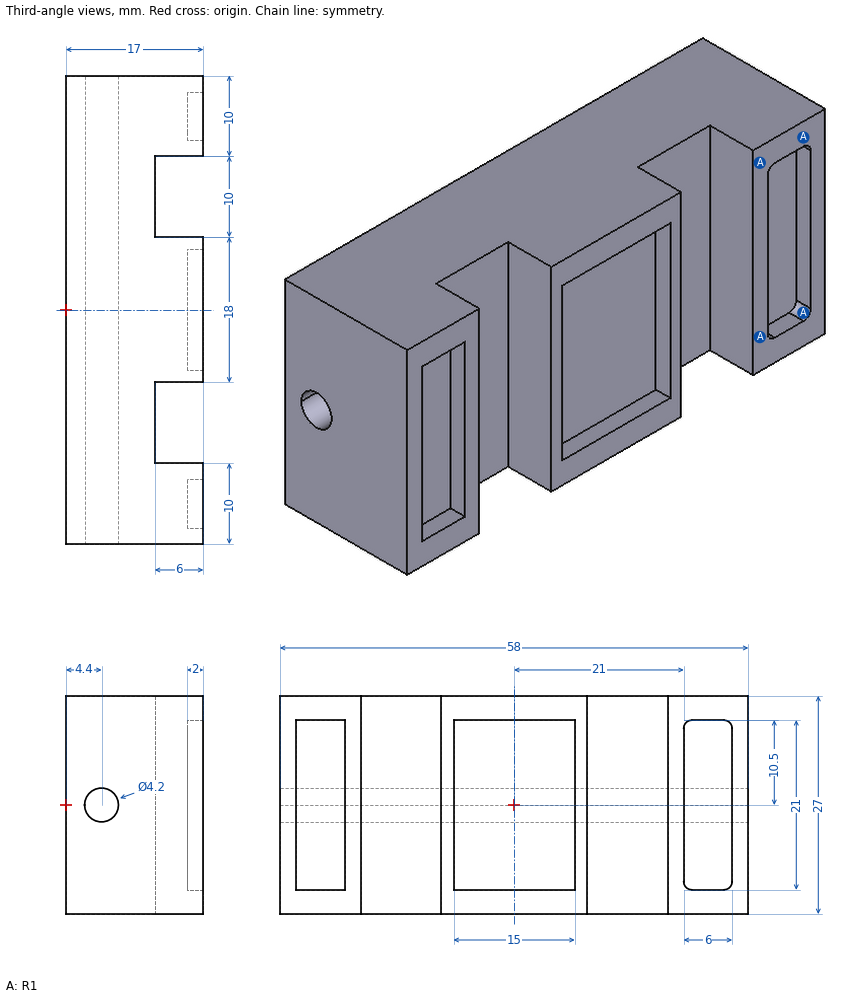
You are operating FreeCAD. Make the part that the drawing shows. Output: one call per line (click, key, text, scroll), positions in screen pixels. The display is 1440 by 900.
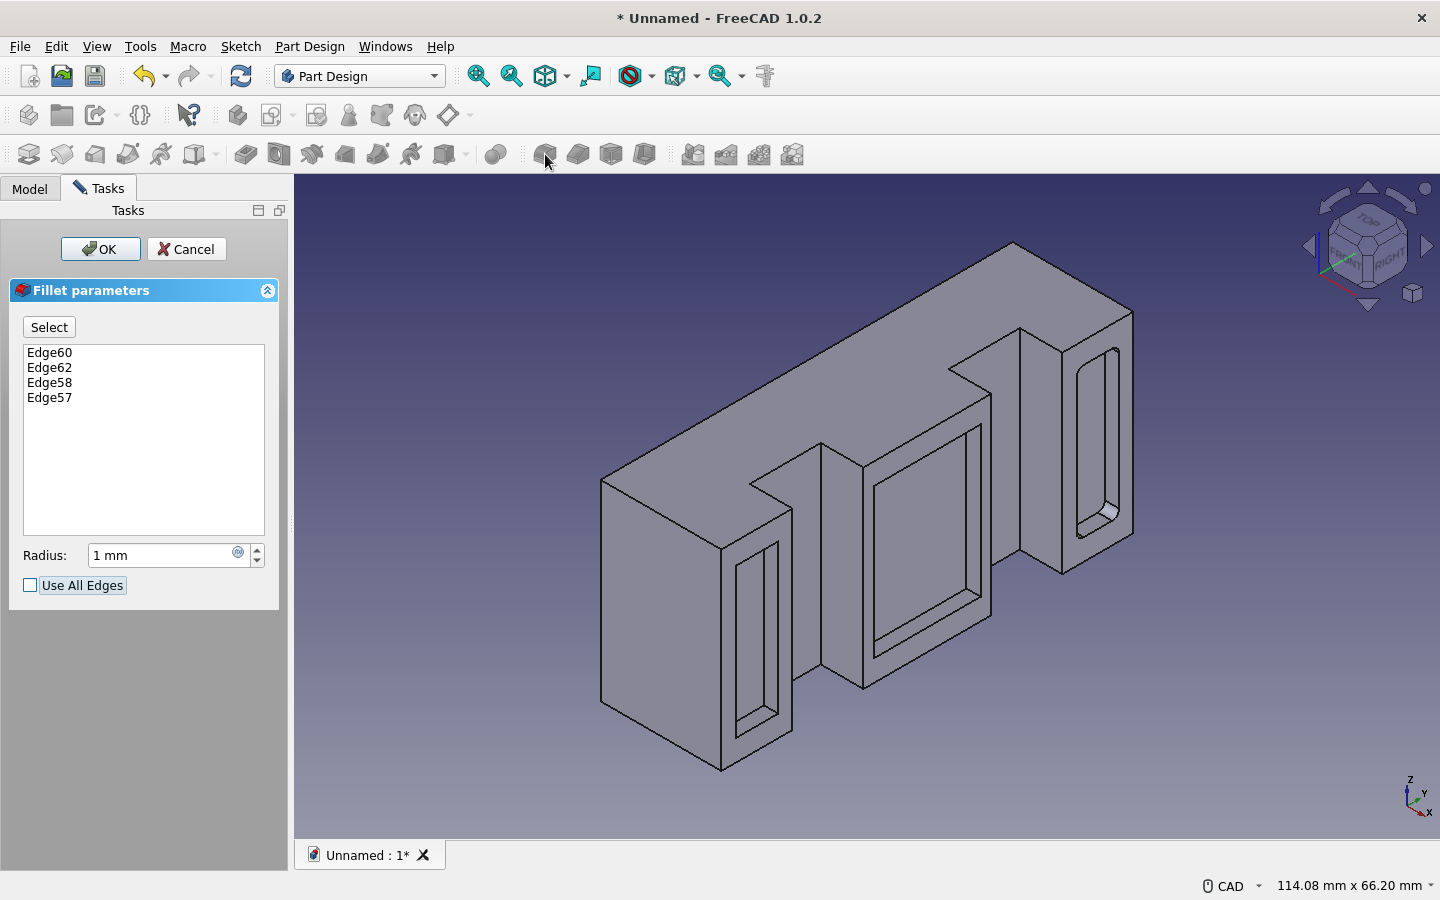
click(101, 249)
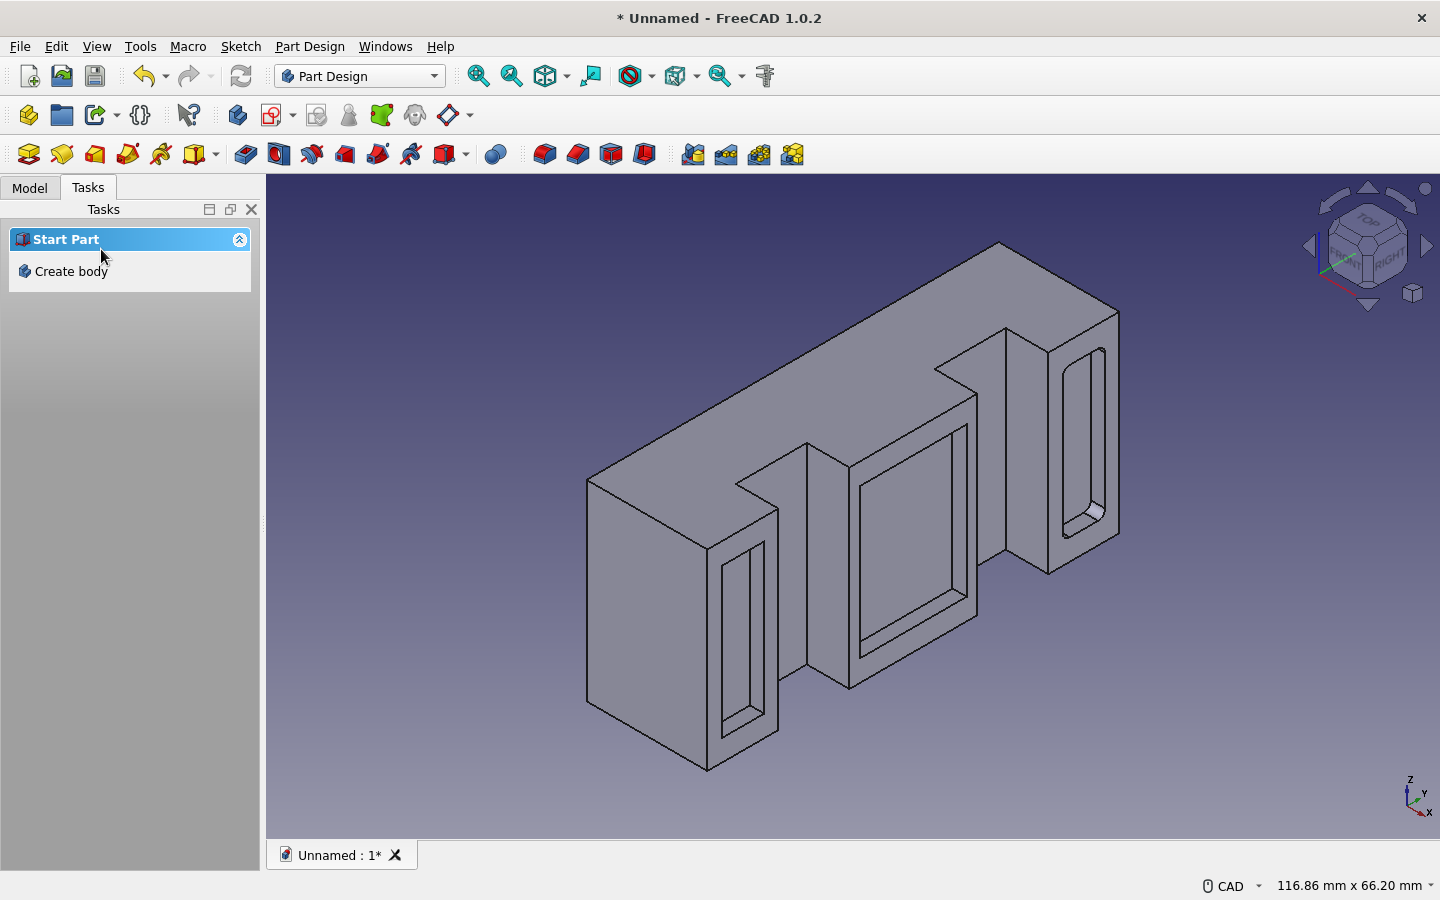
key(4)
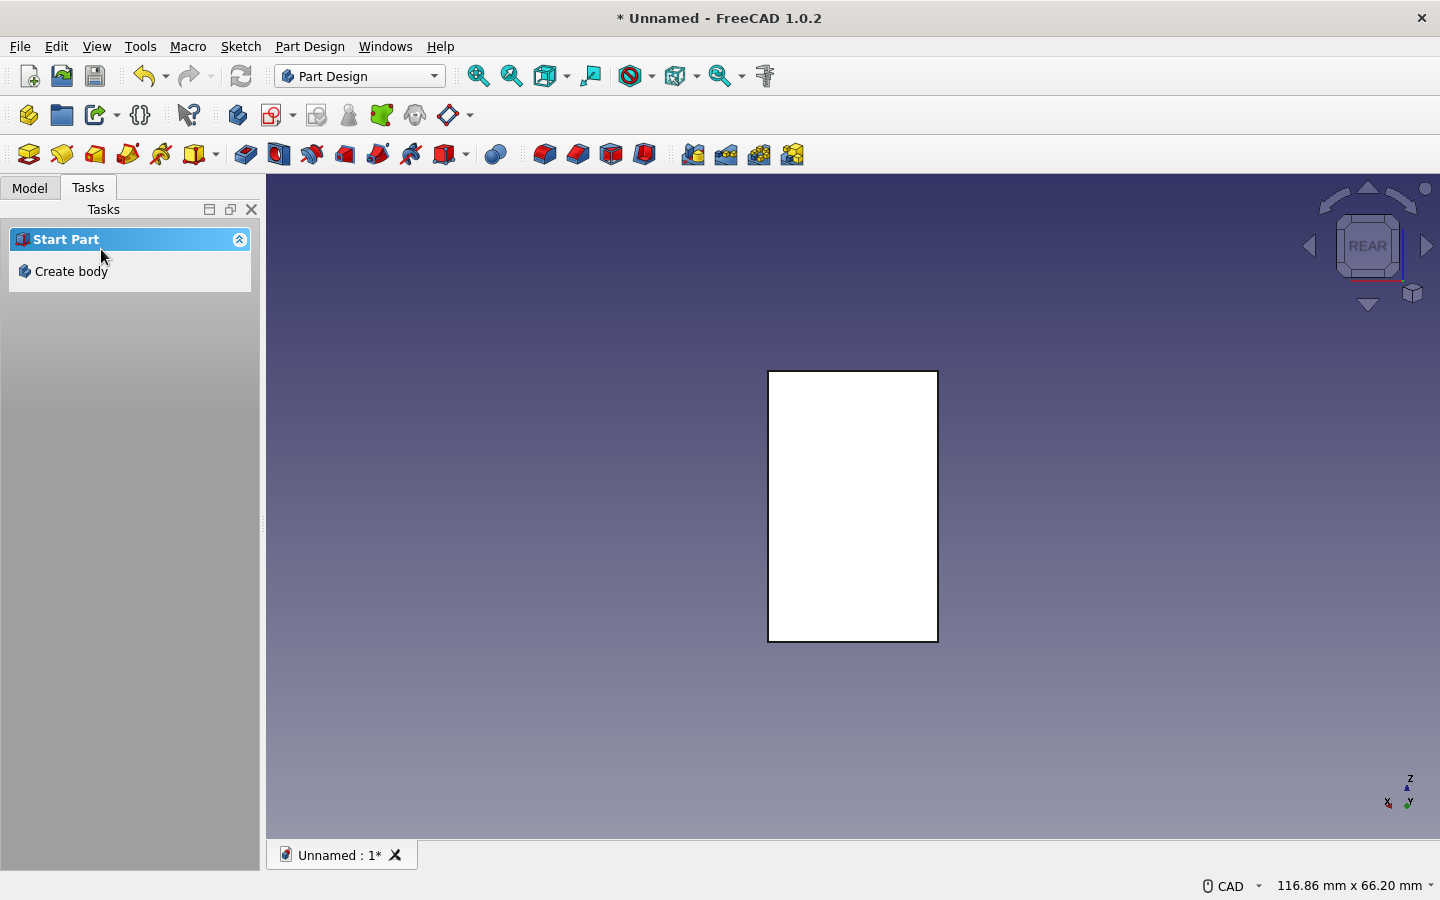
key(v)
key(f)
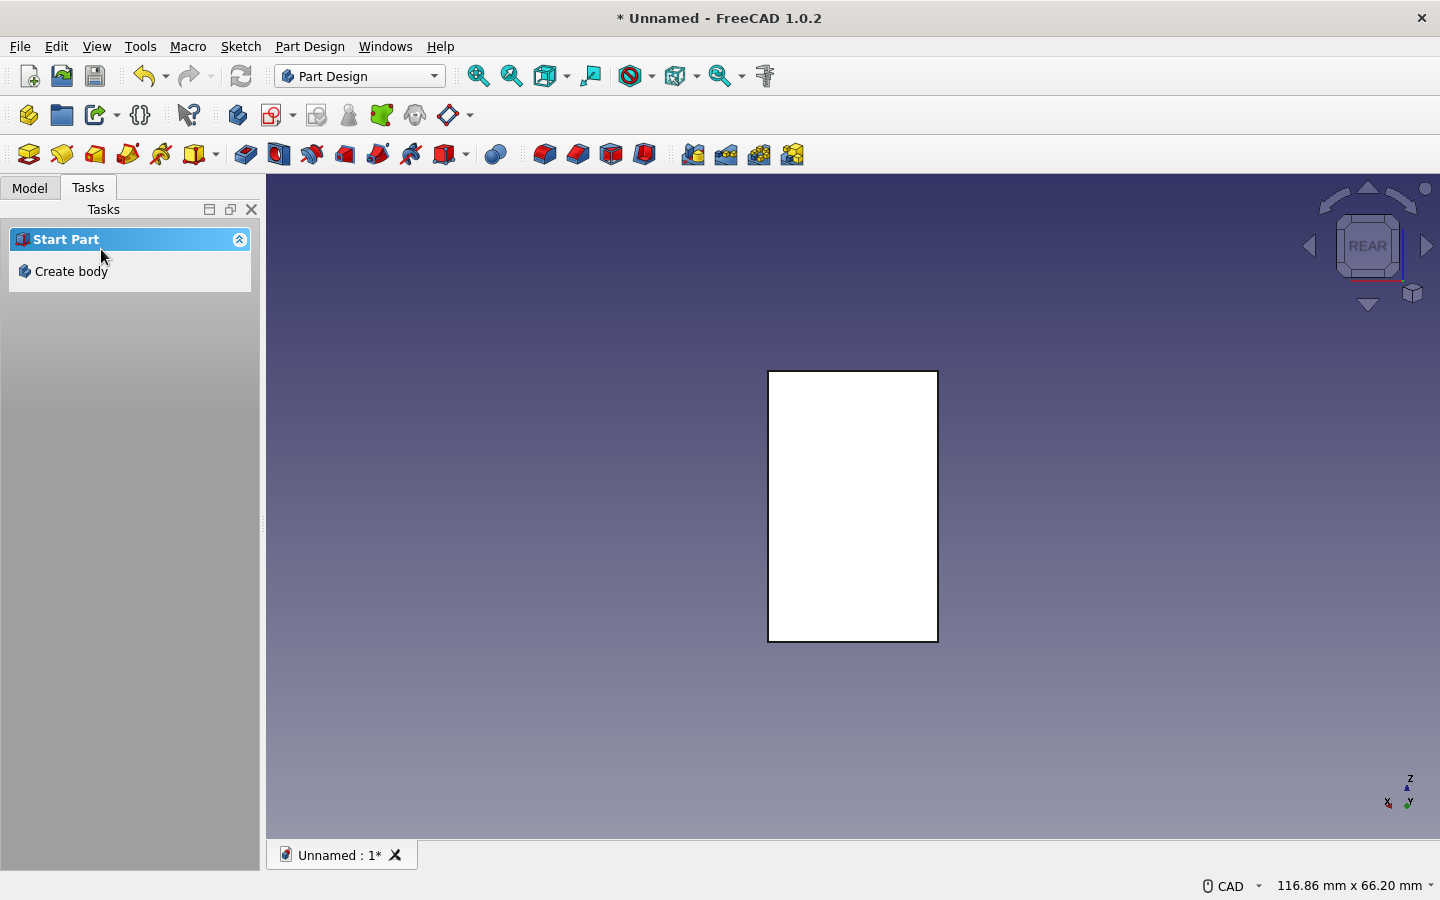
click(853, 467)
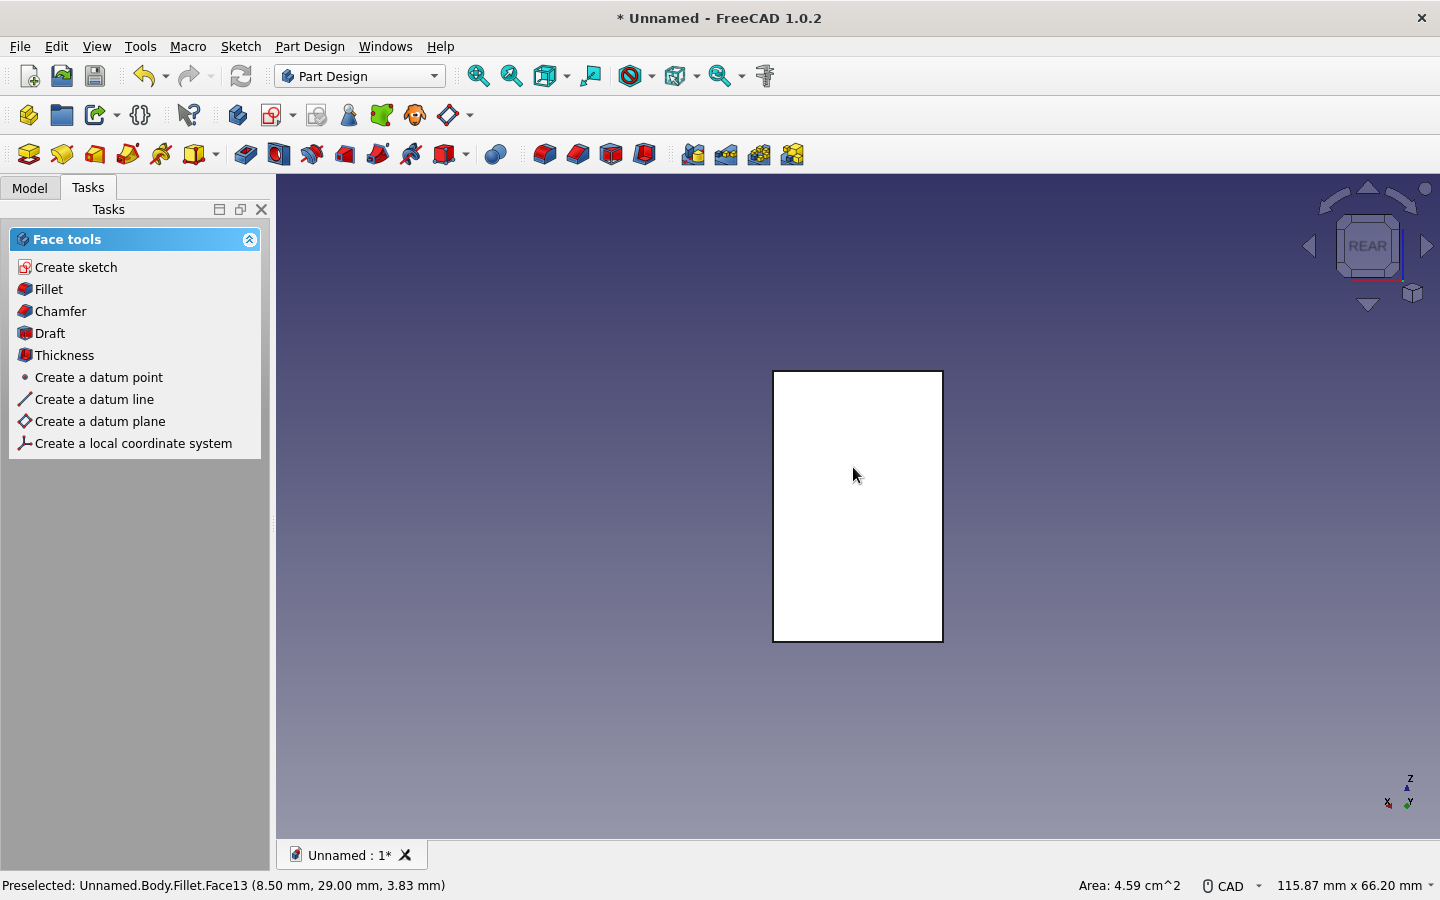
click(270, 116)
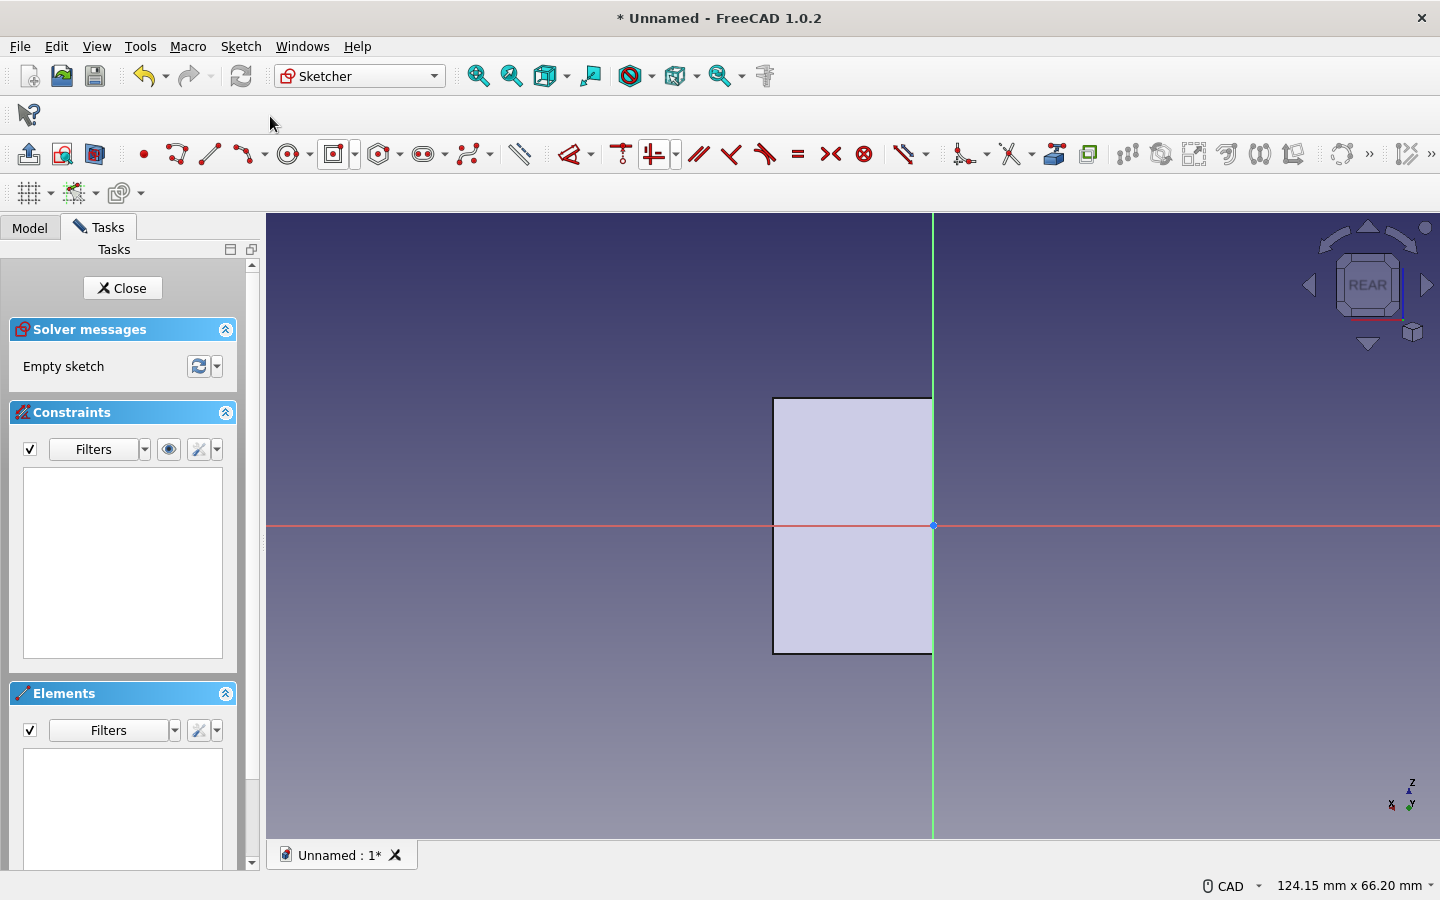
scroll(914, 526, up, 12)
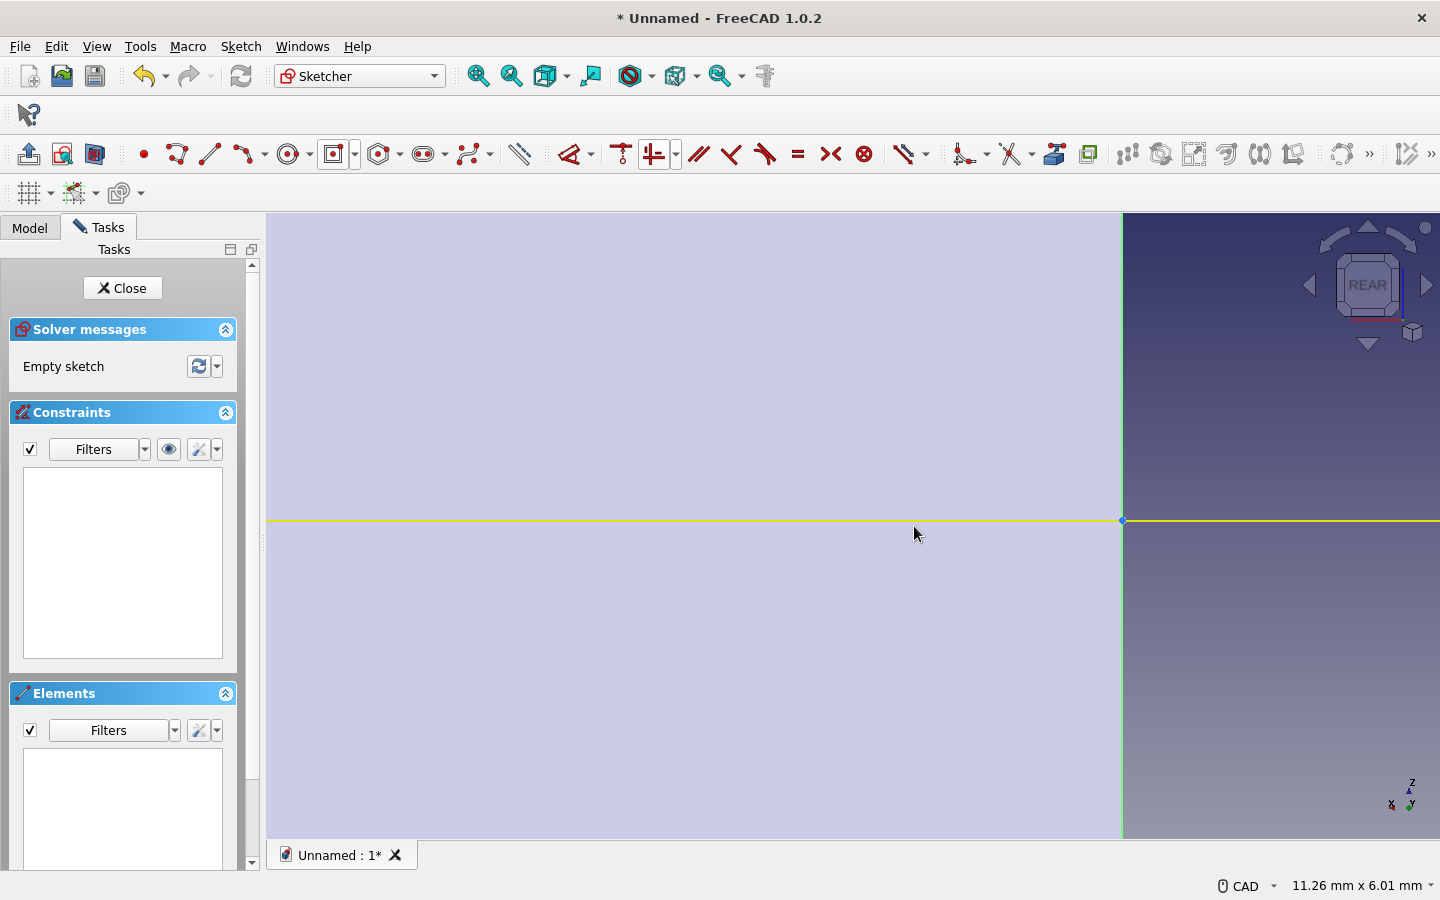
click(288, 154)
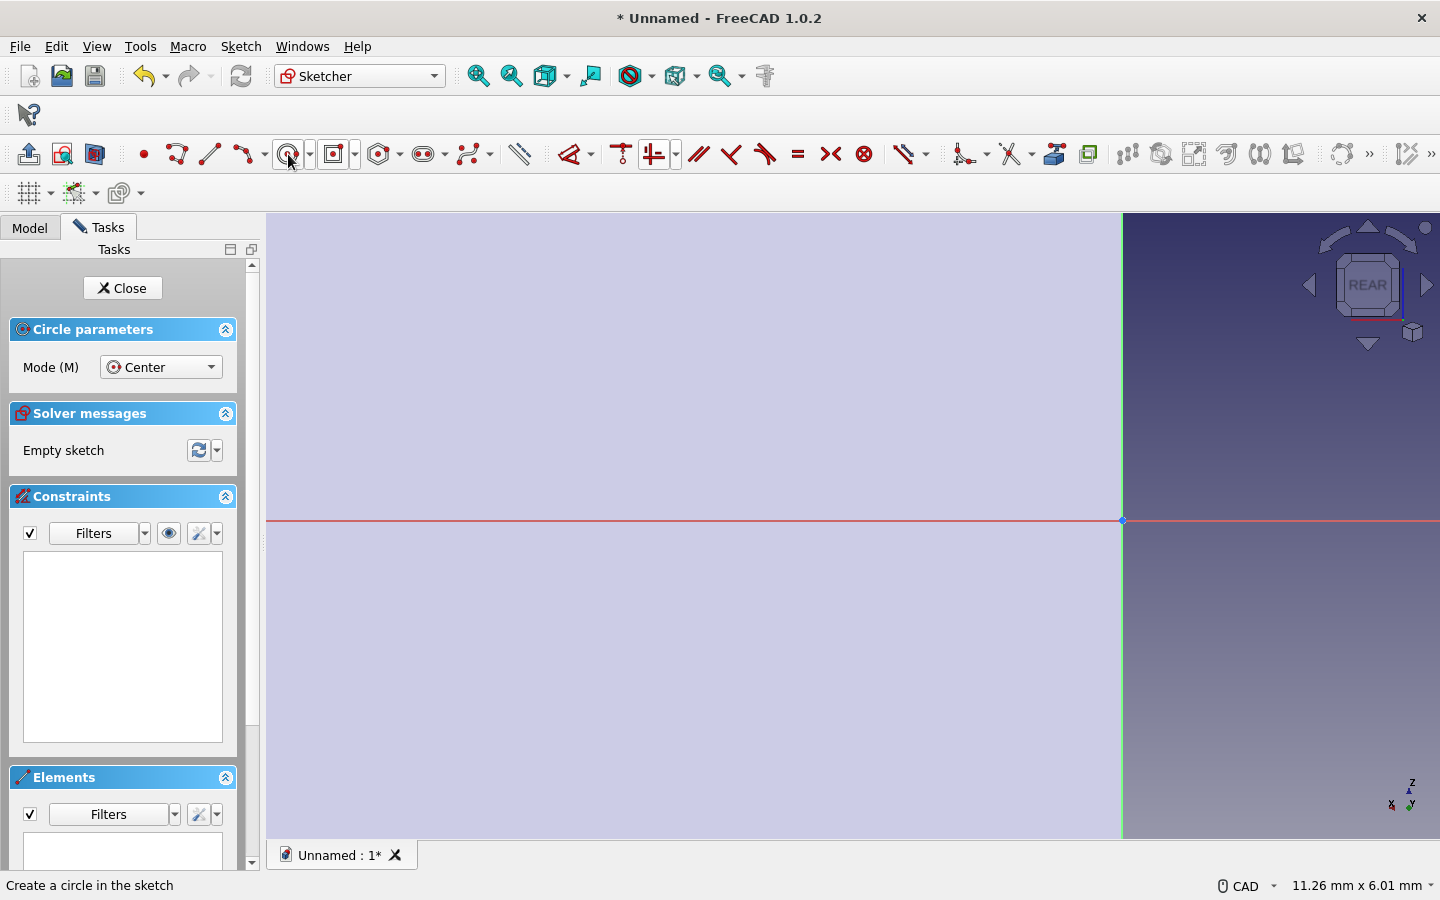
click(663, 521)
click(818, 366)
key(Escape)